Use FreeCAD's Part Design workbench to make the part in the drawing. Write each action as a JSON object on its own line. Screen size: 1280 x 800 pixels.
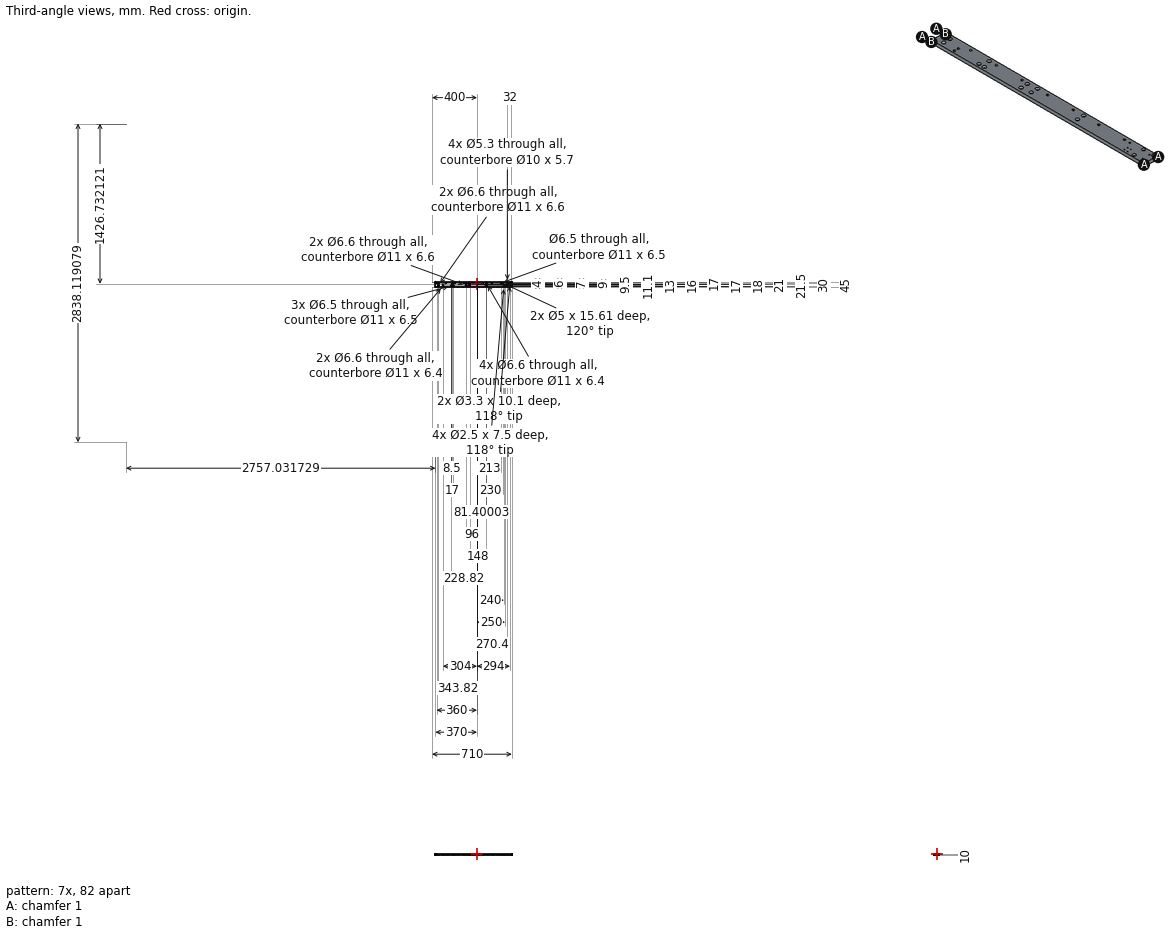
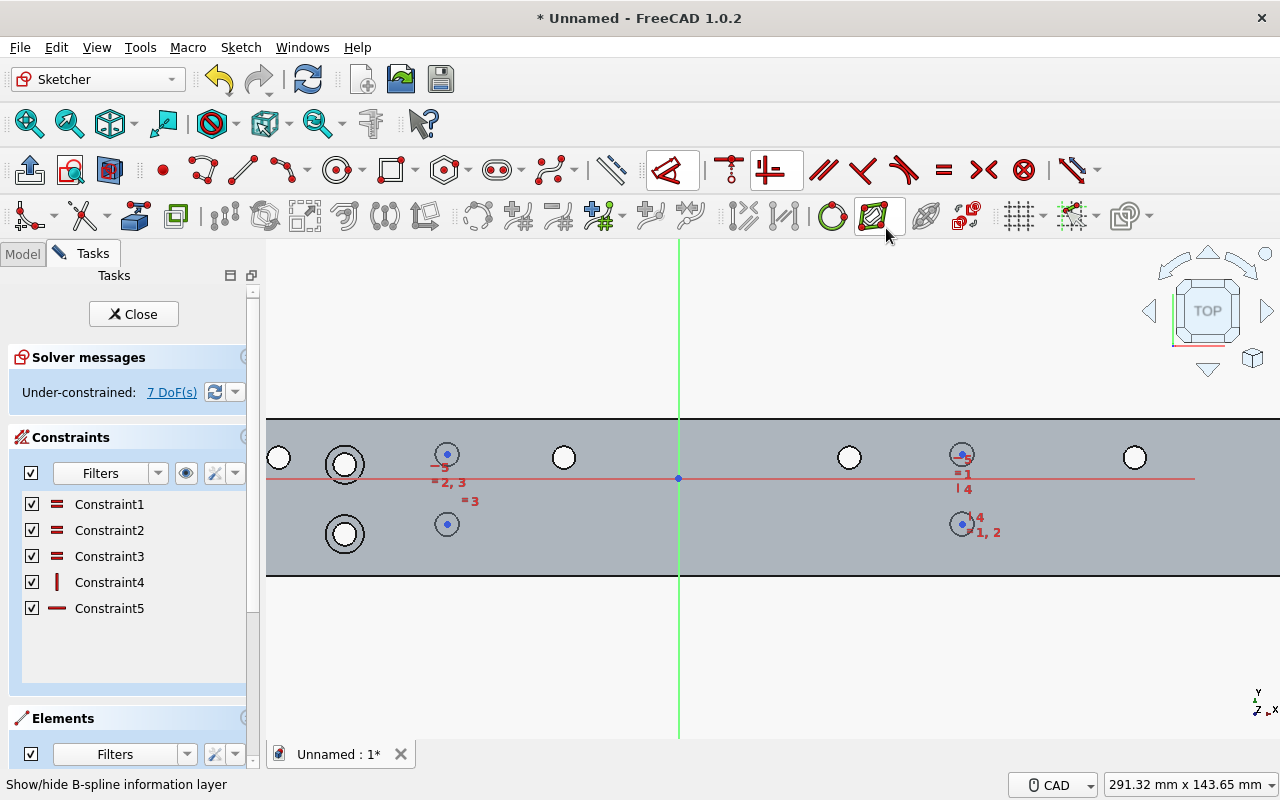
{"action": "left_click", "coordinate": [447, 454]}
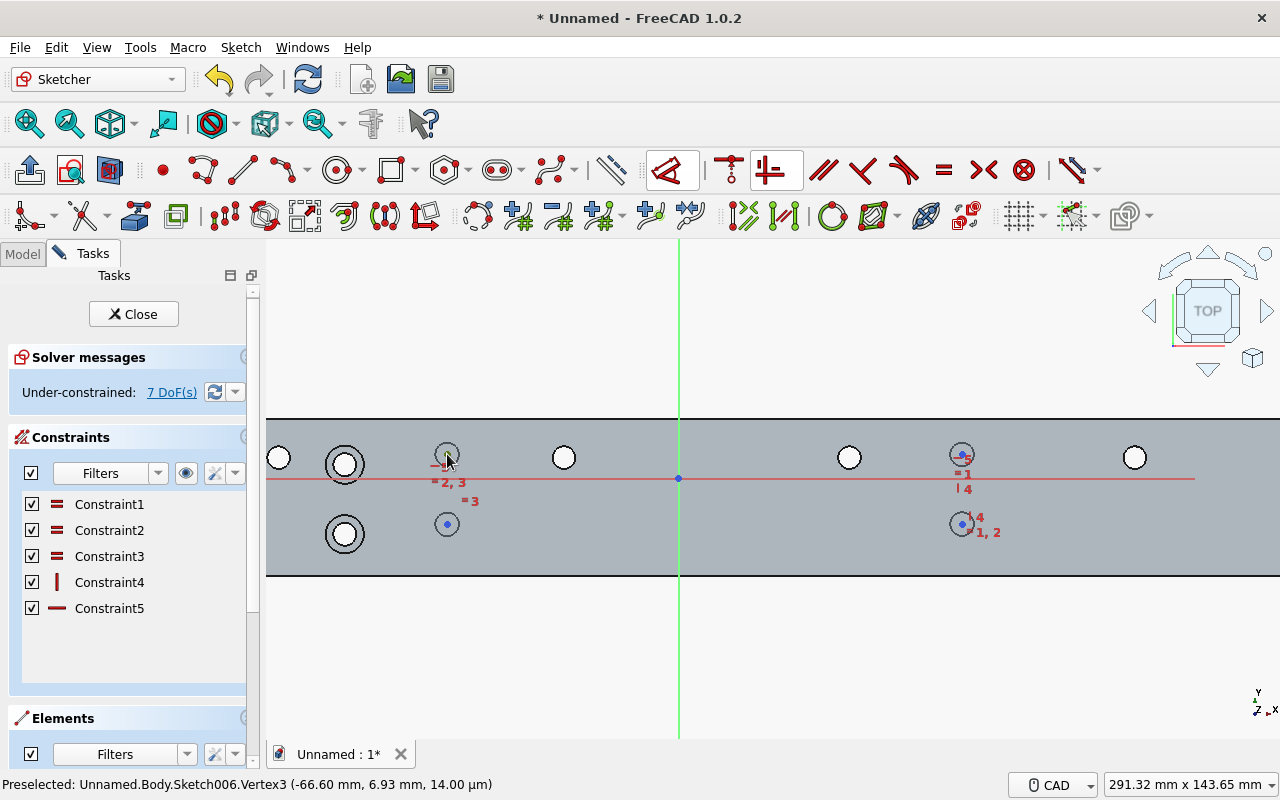
{"action": "left_click", "coordinate": [447, 524]}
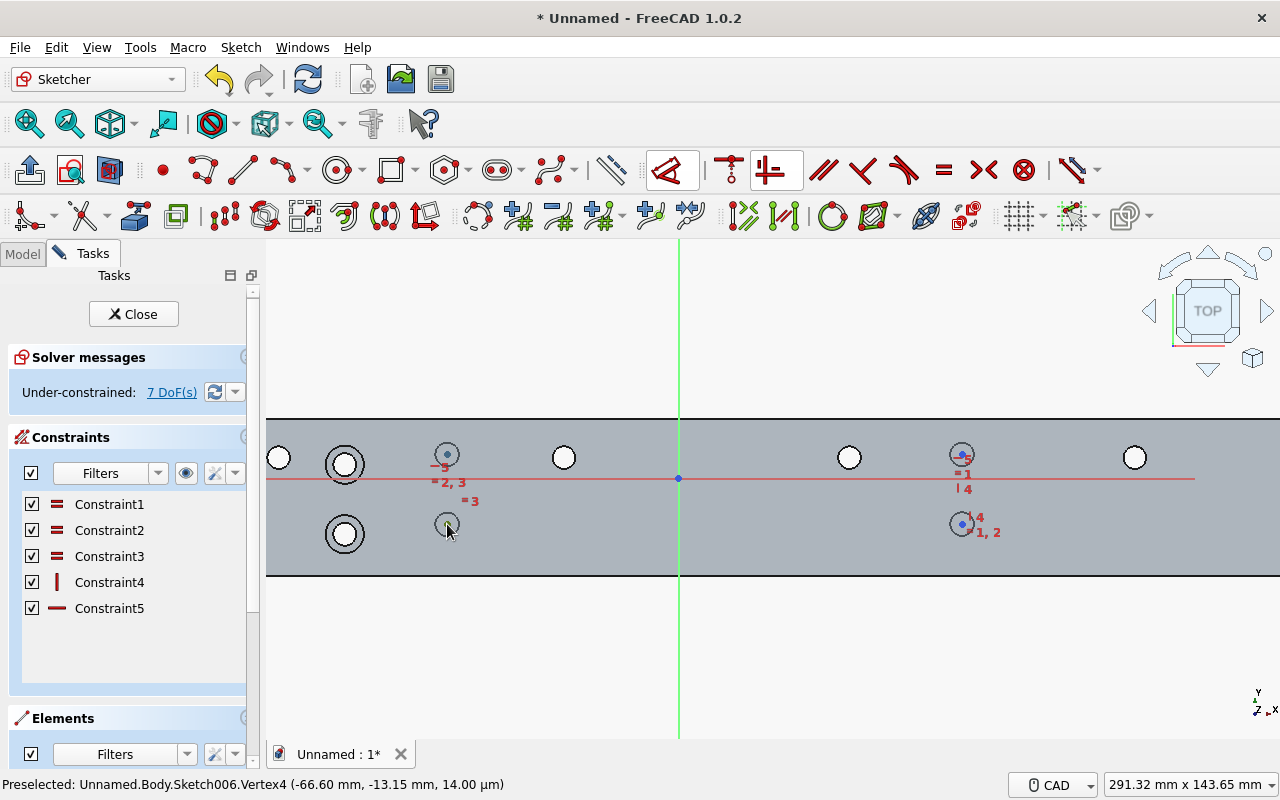
{"action": "left_click", "coordinate": [798, 170]}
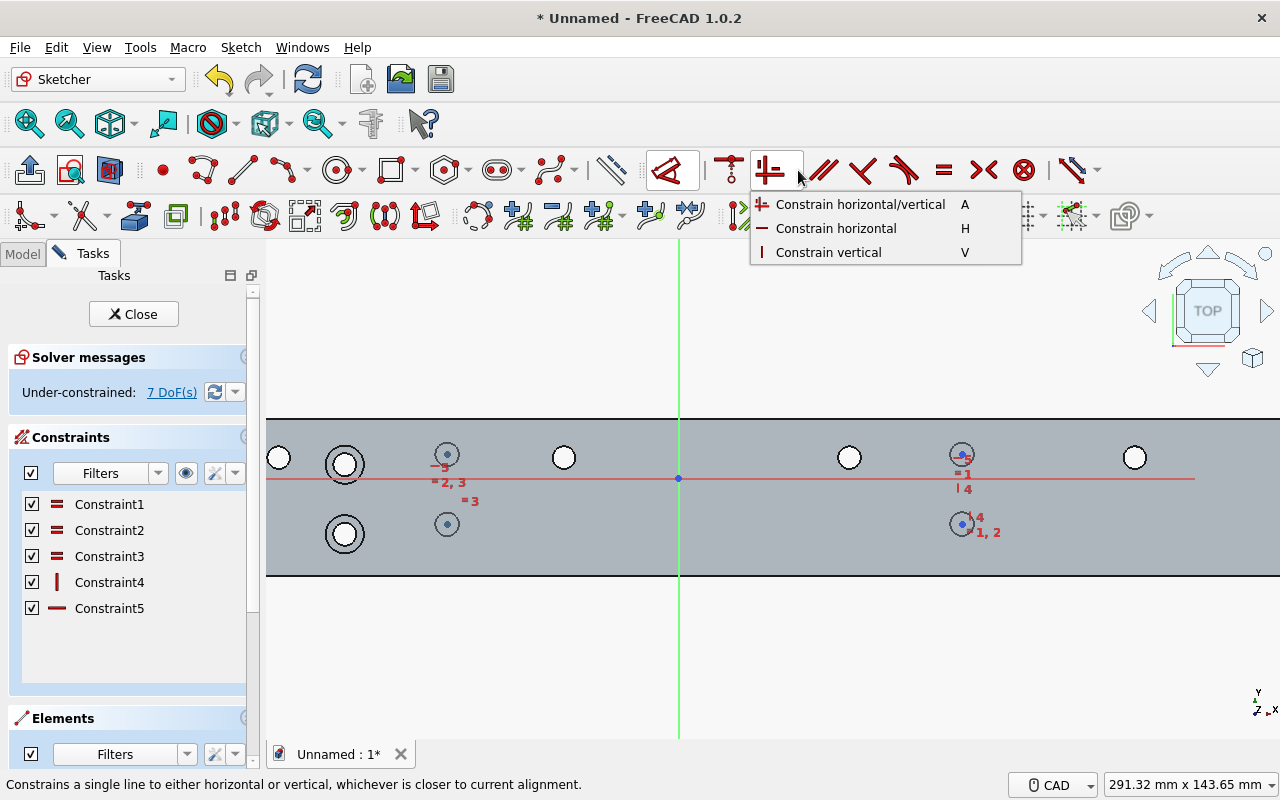
{"action": "left_click", "coordinate": [886, 252]}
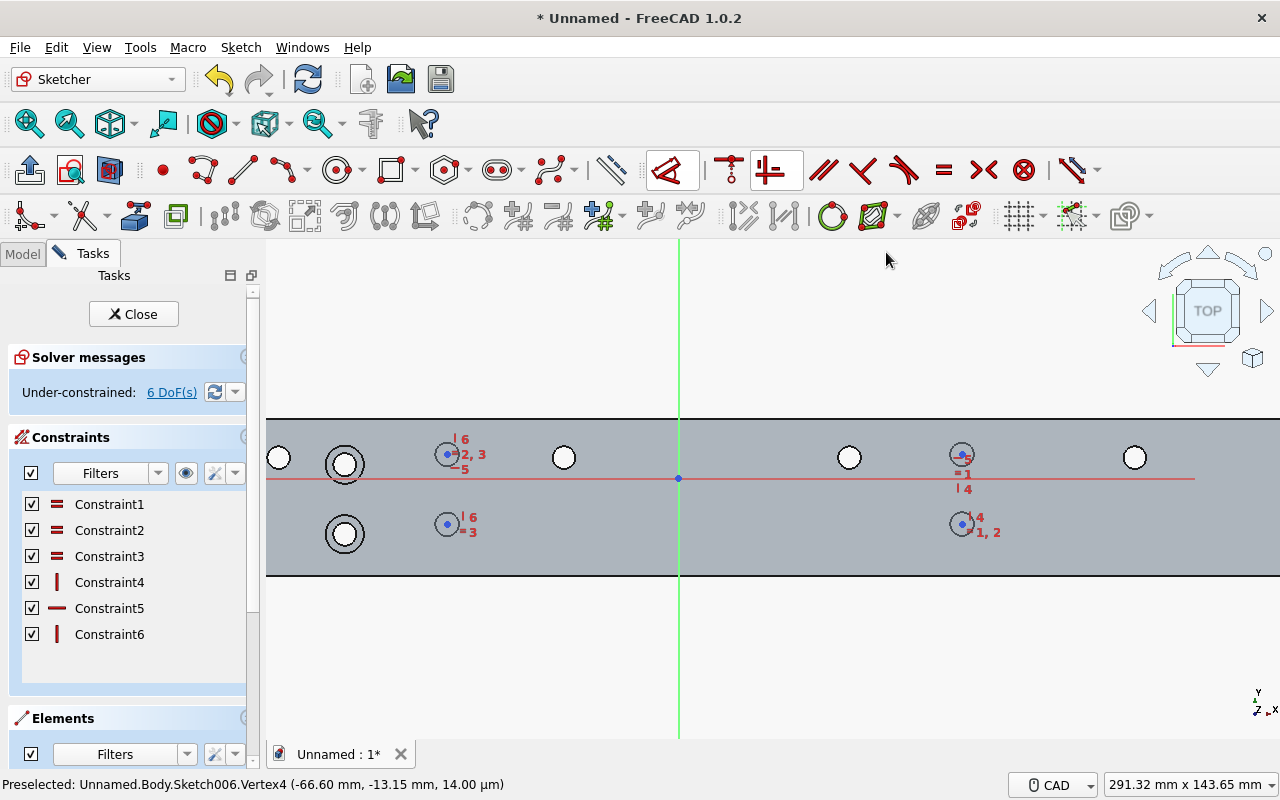
{"action": "left_click", "coordinate": [962, 524]}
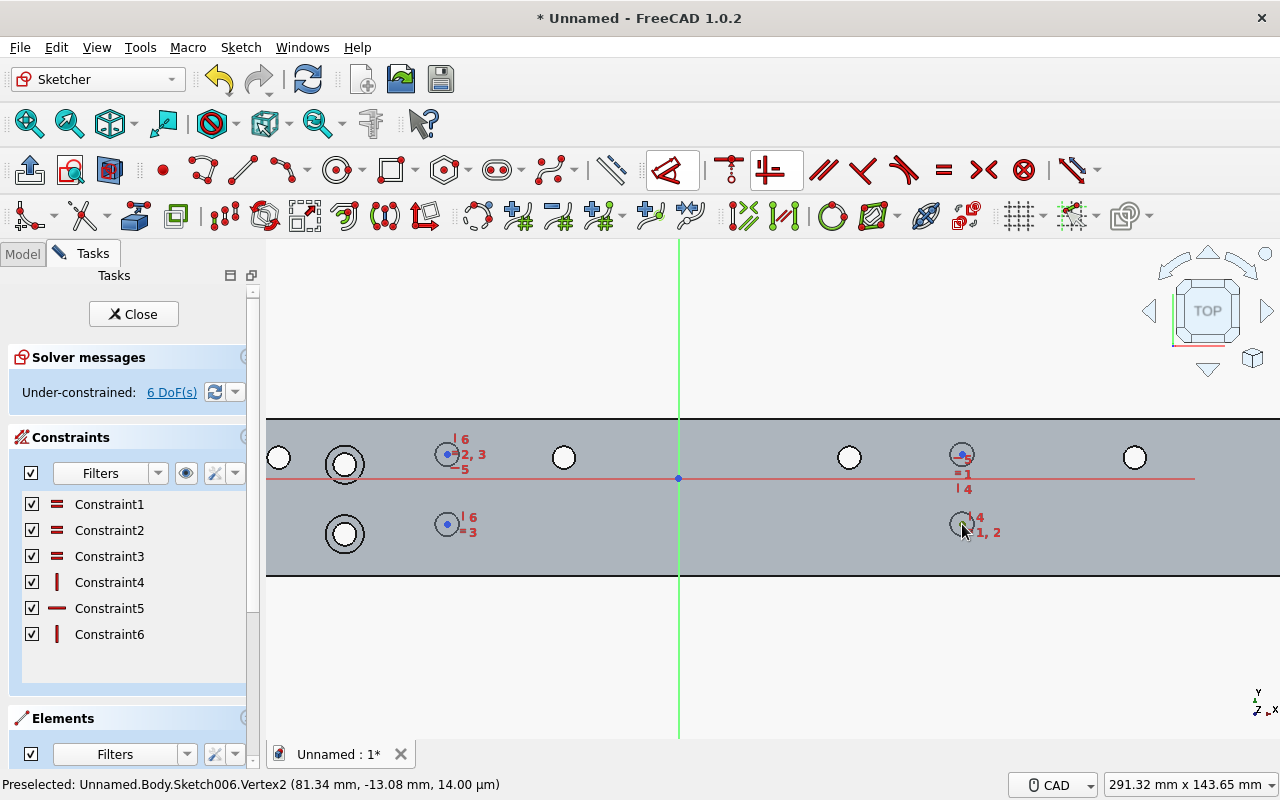
{"action": "left_click", "coordinate": [447, 524]}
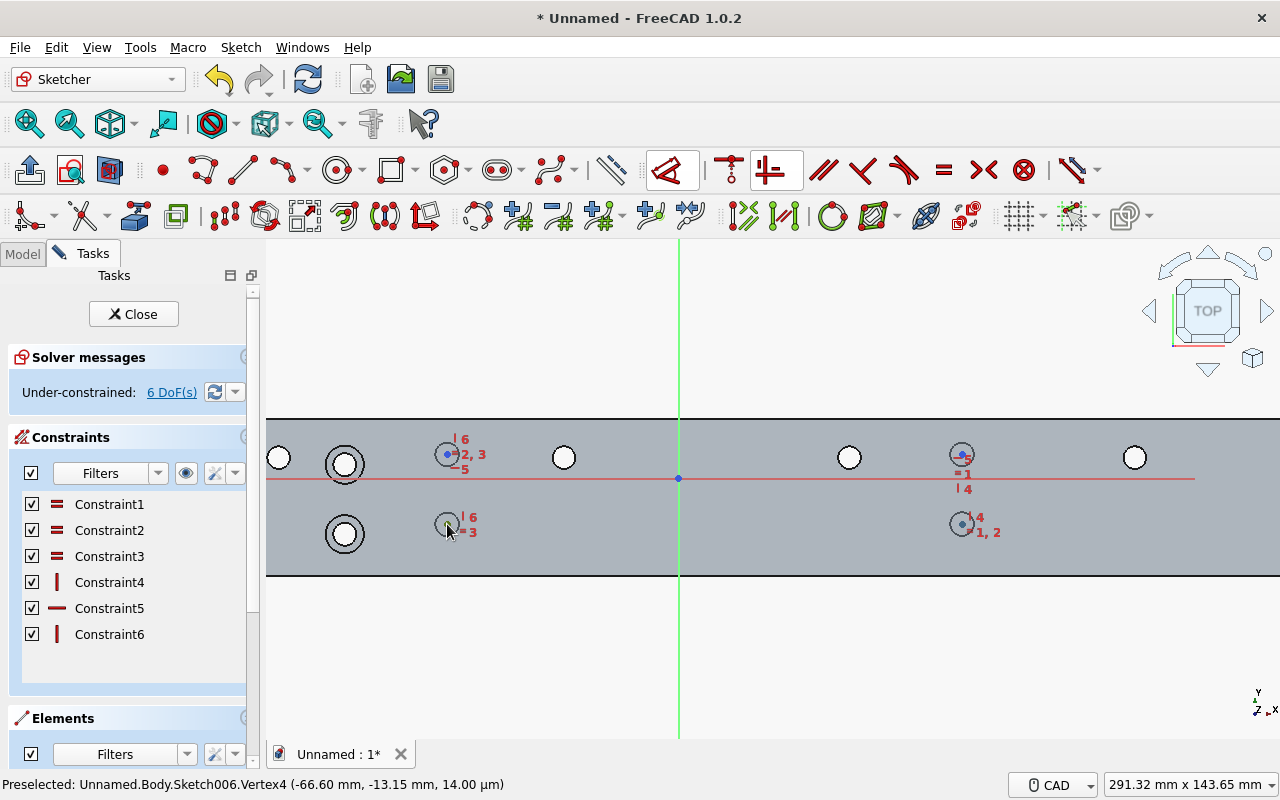
{"action": "left_click", "coordinate": [798, 170]}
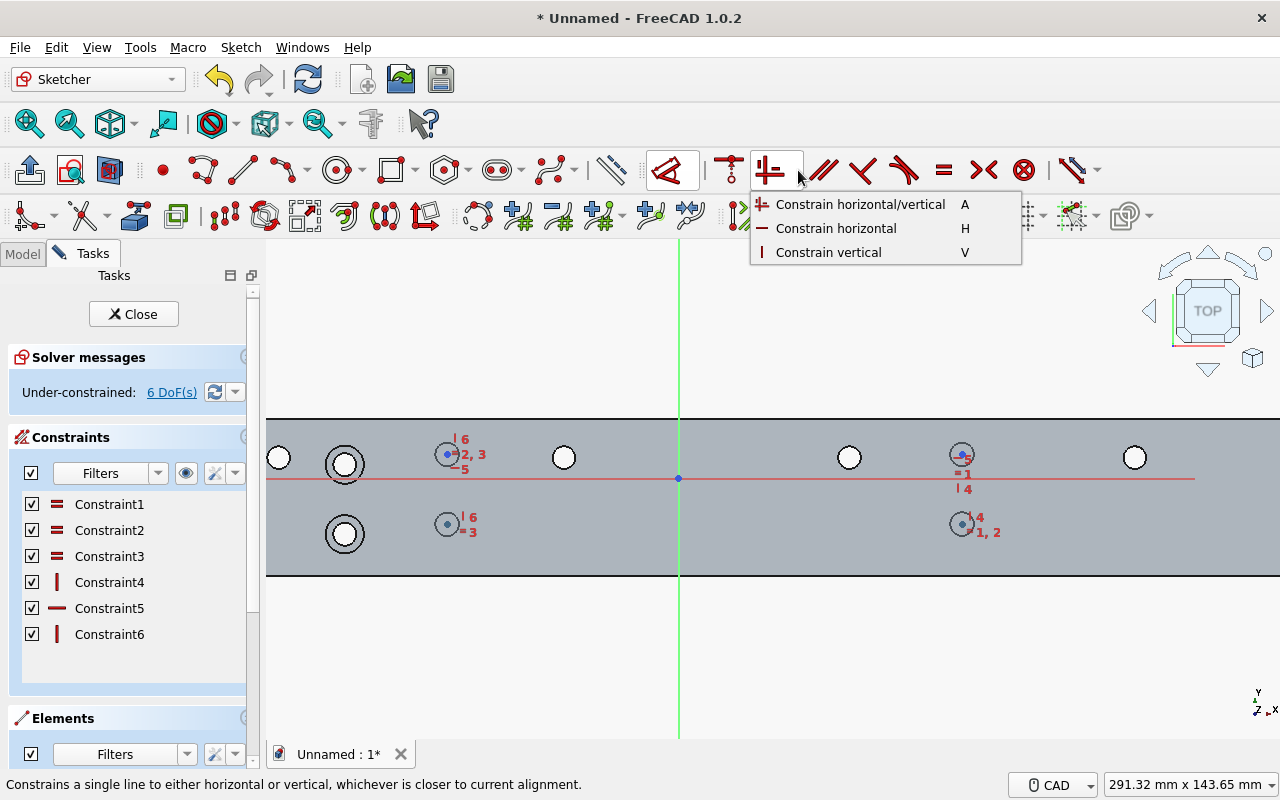
{"action": "left_click", "coordinate": [886, 228]}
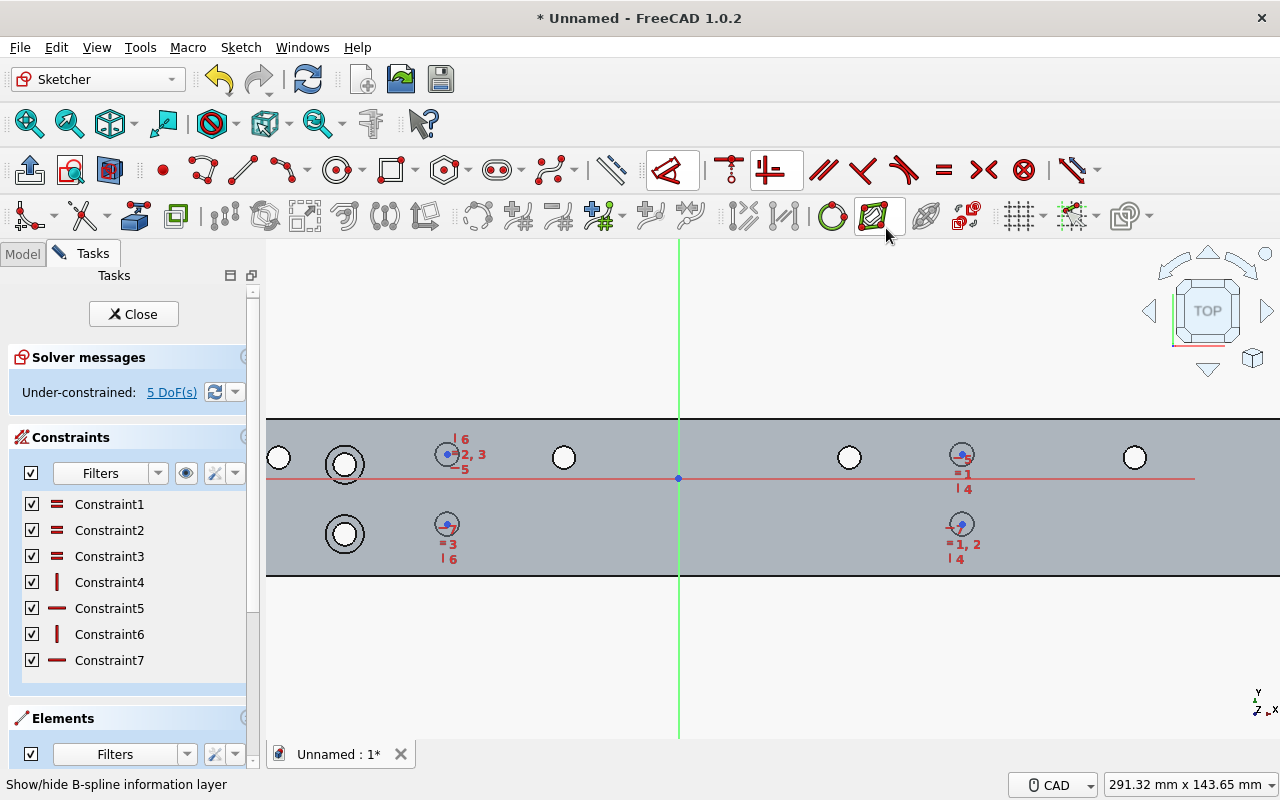
{"action": "scroll", "coordinate": [970, 446], "scroll_direction": "up", "scroll_amount": 3}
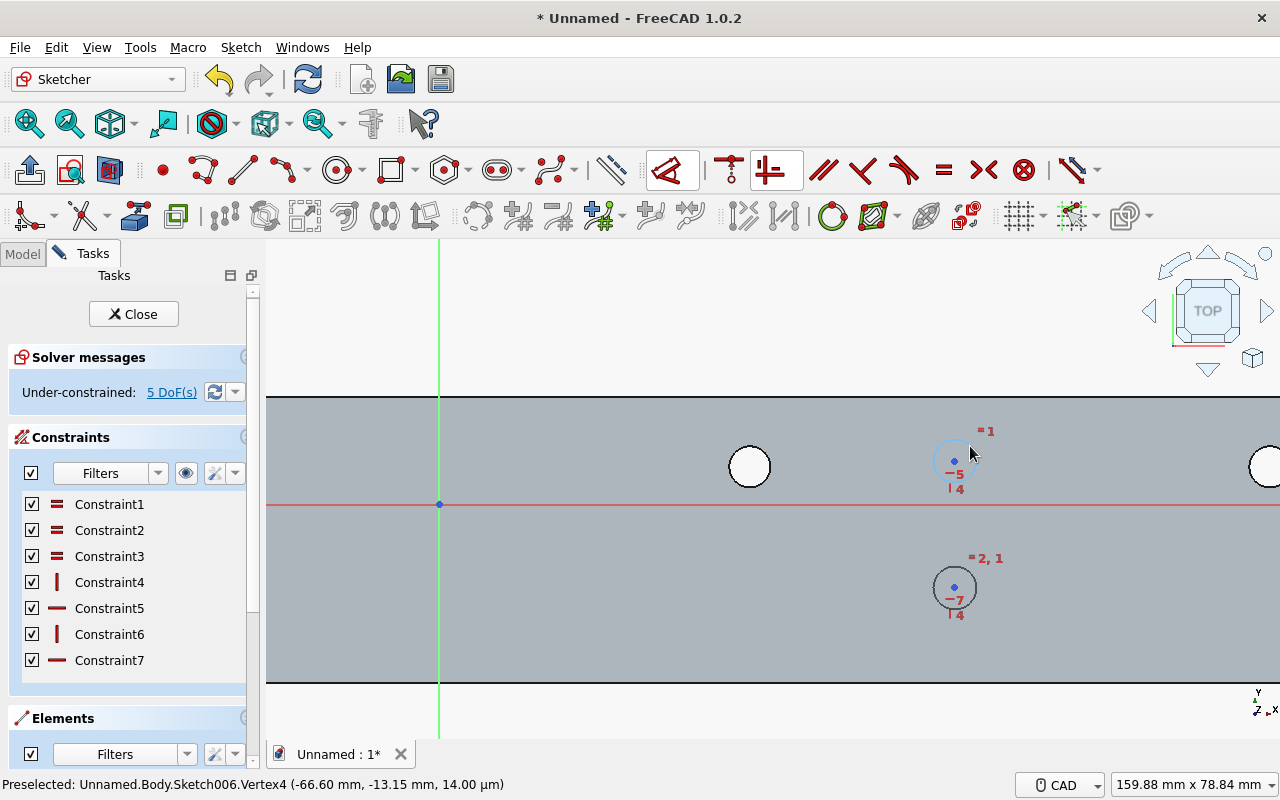
{"action": "left_click", "coordinate": [970, 446]}